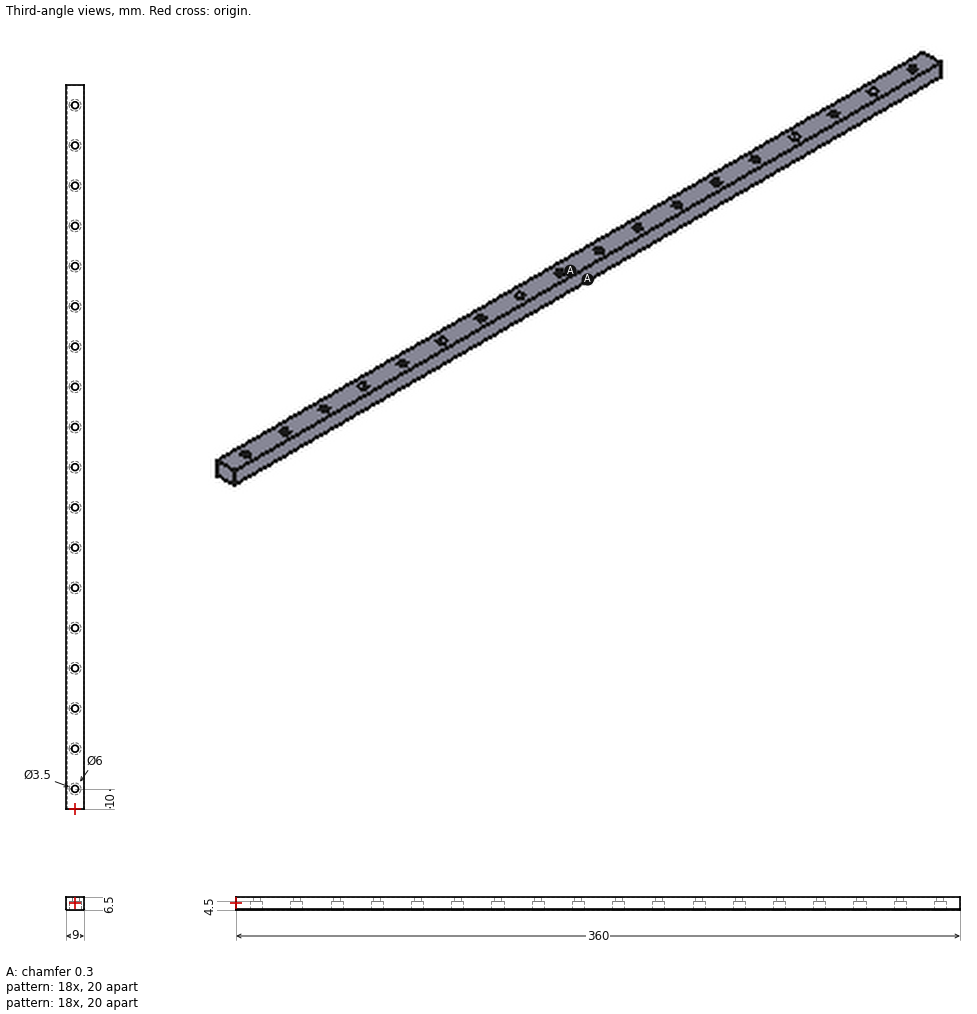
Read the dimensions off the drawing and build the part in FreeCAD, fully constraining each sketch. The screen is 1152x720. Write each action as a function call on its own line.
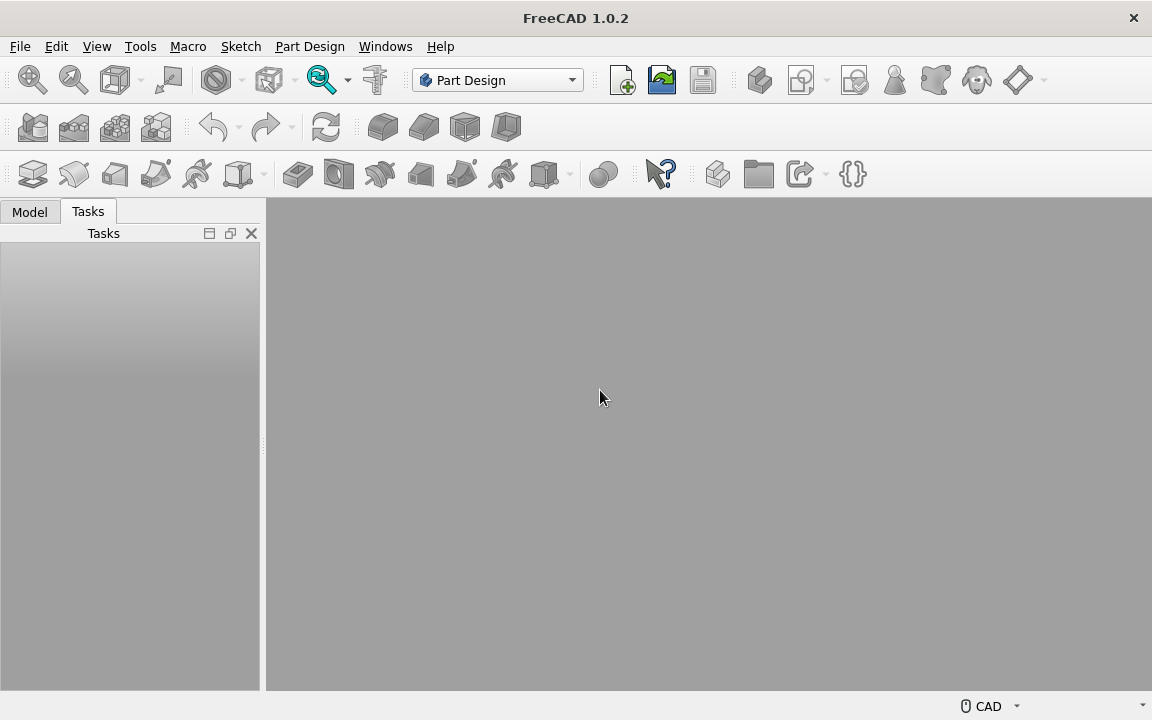
click(621, 80)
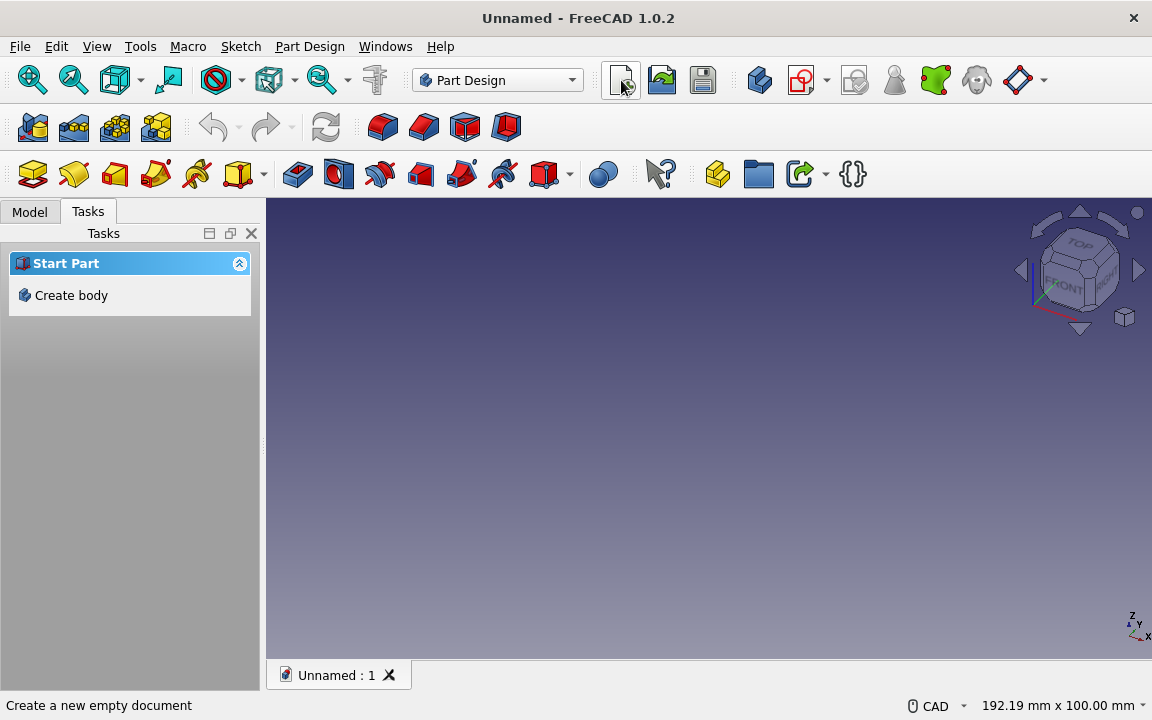
click(800, 80)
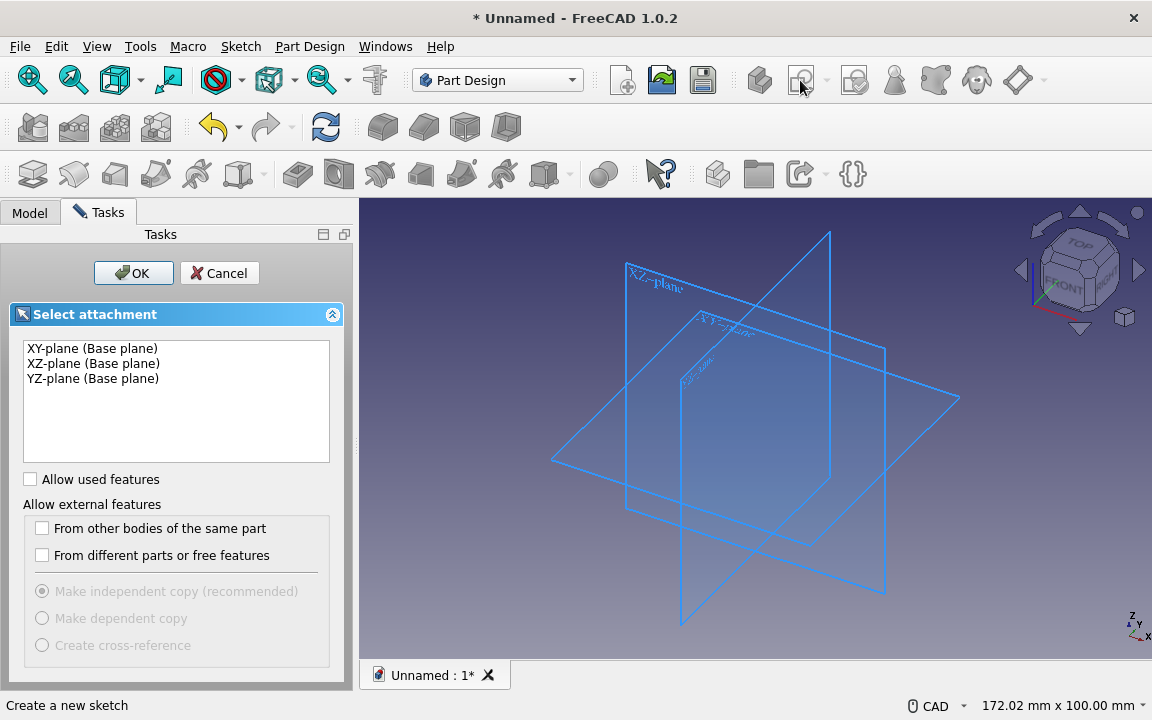
click(84, 364)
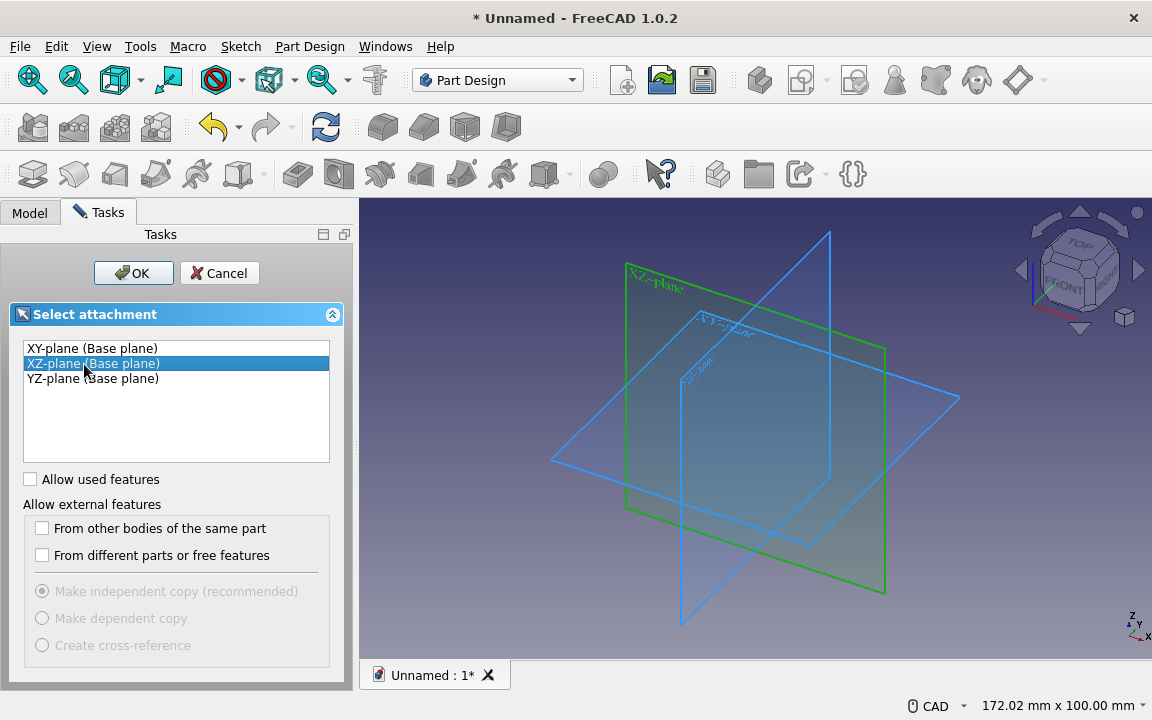
click(134, 273)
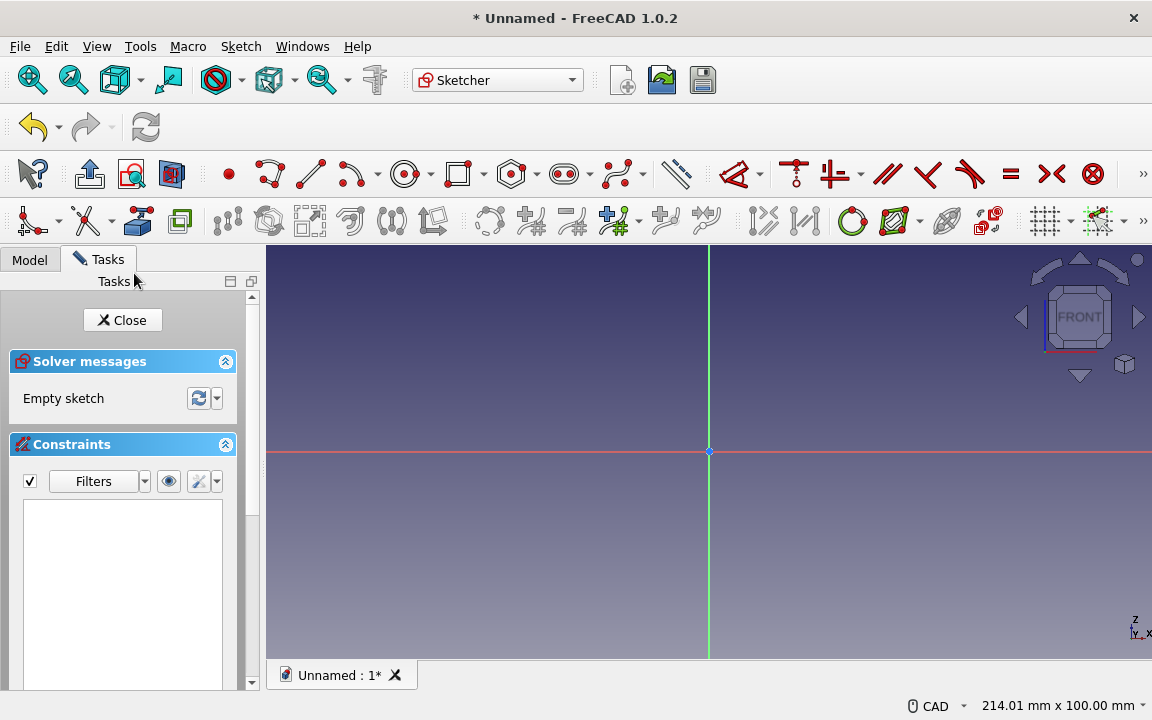
scroll(718, 452, up, 11)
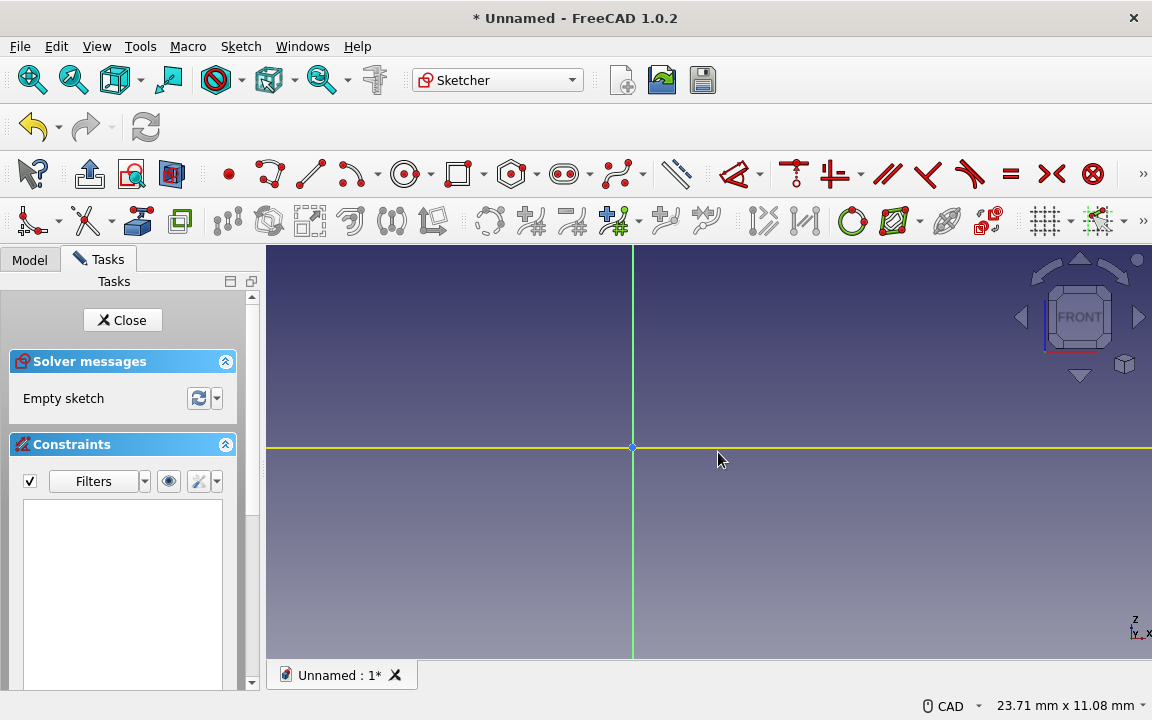
key(g)
key(v)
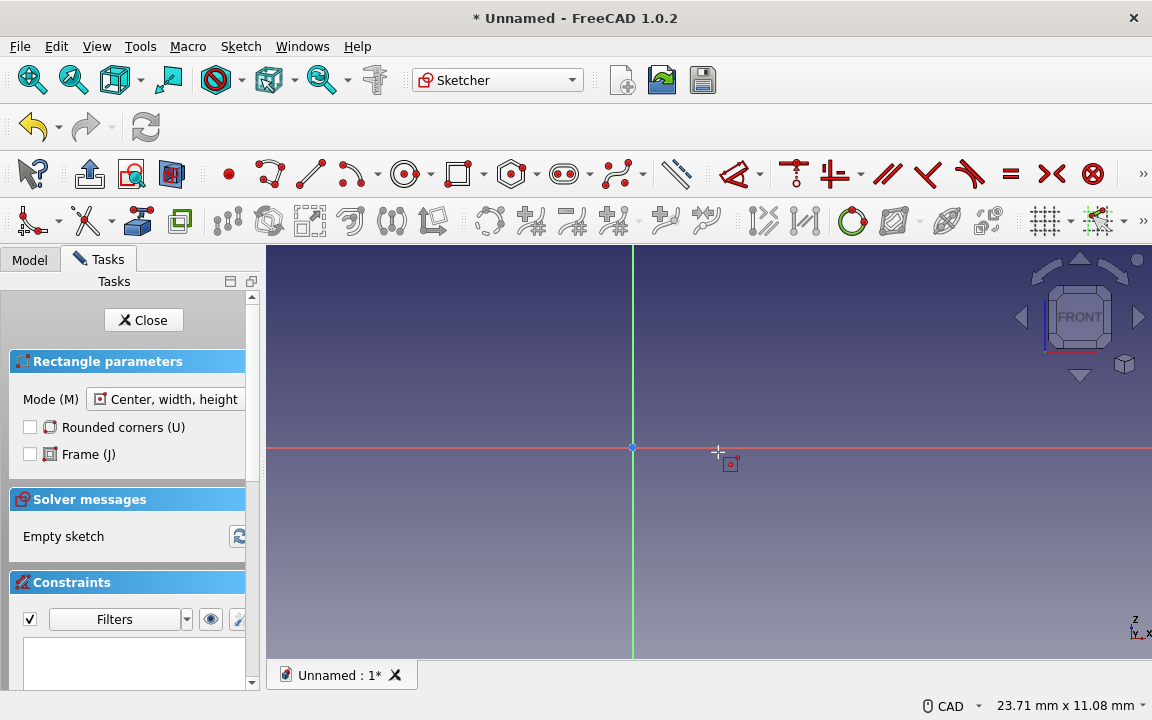
click(633, 448)
move(801, 327)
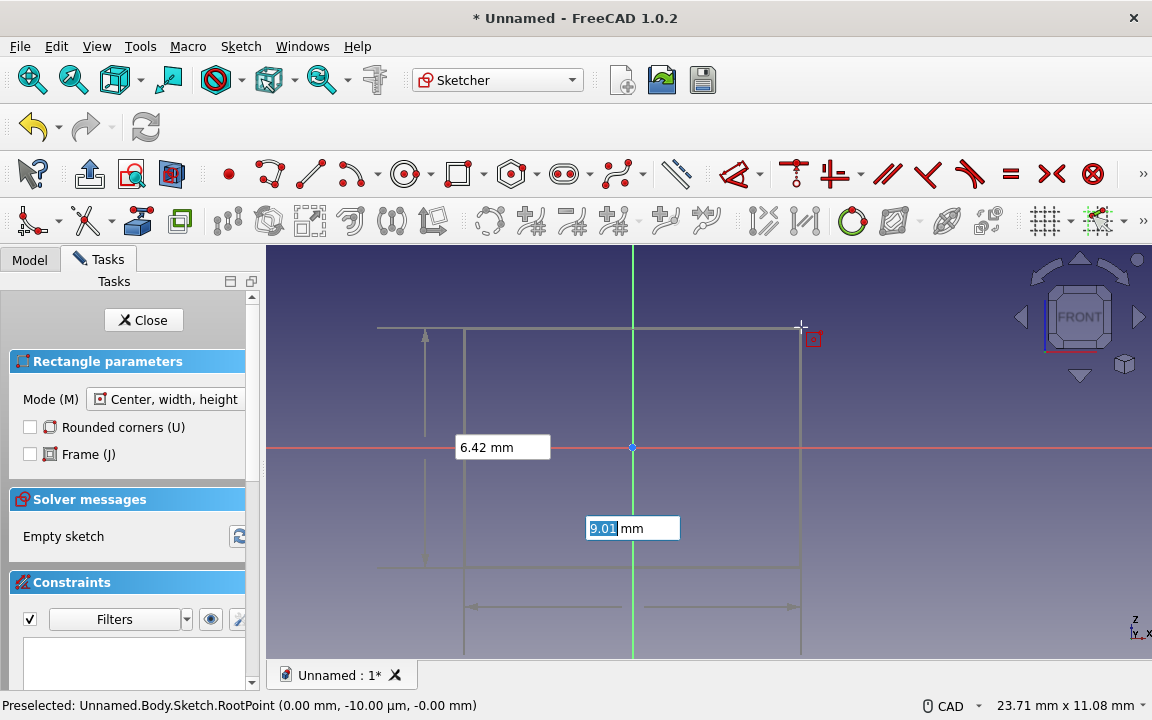
text(9)
key(Tab)
text(6.5)
key(Return)
key(Escape)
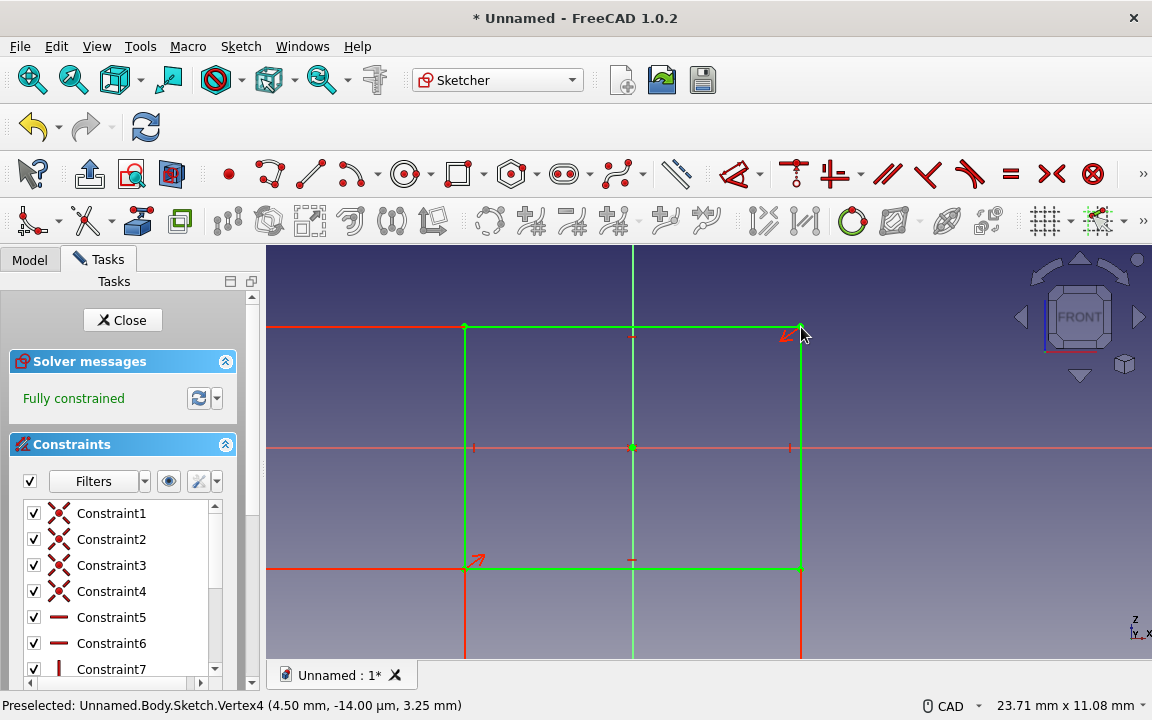
click(123, 320)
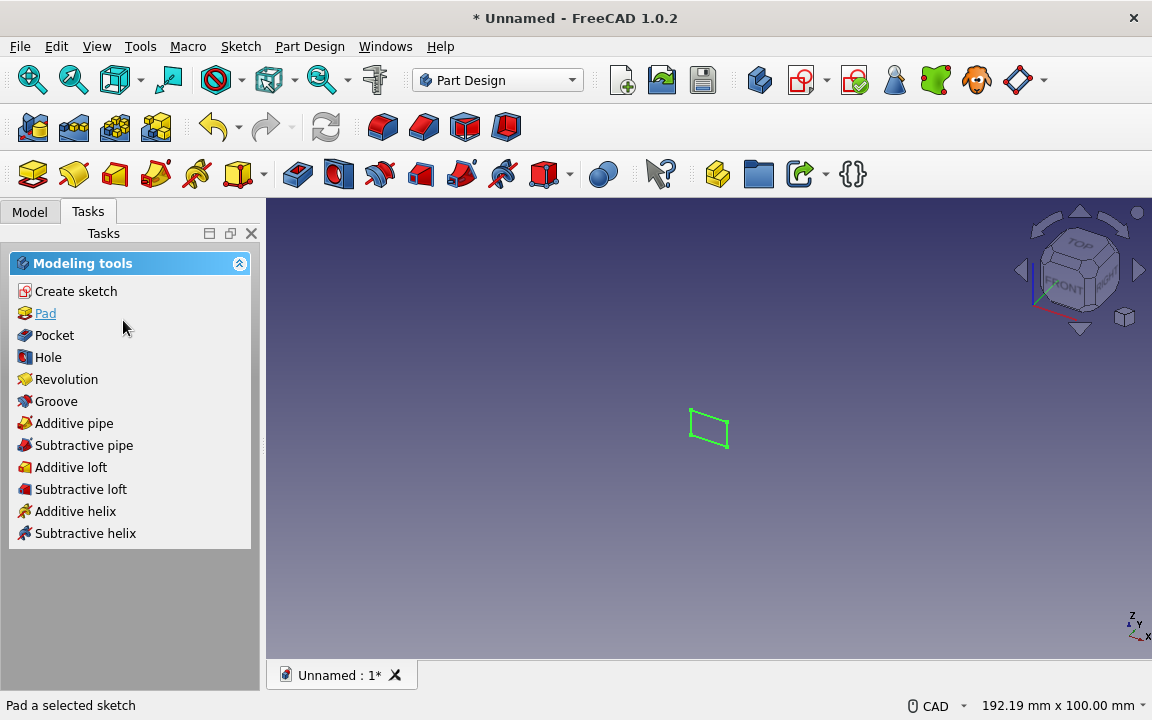
click(33, 174)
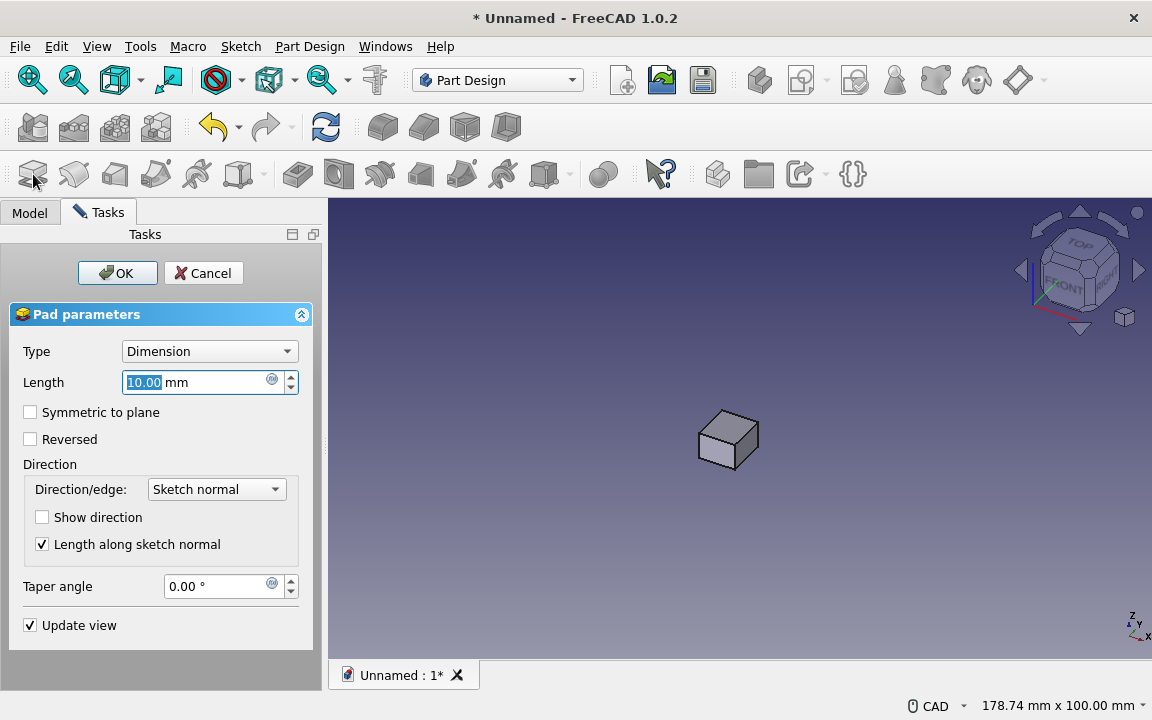
text(360)
key(Tab)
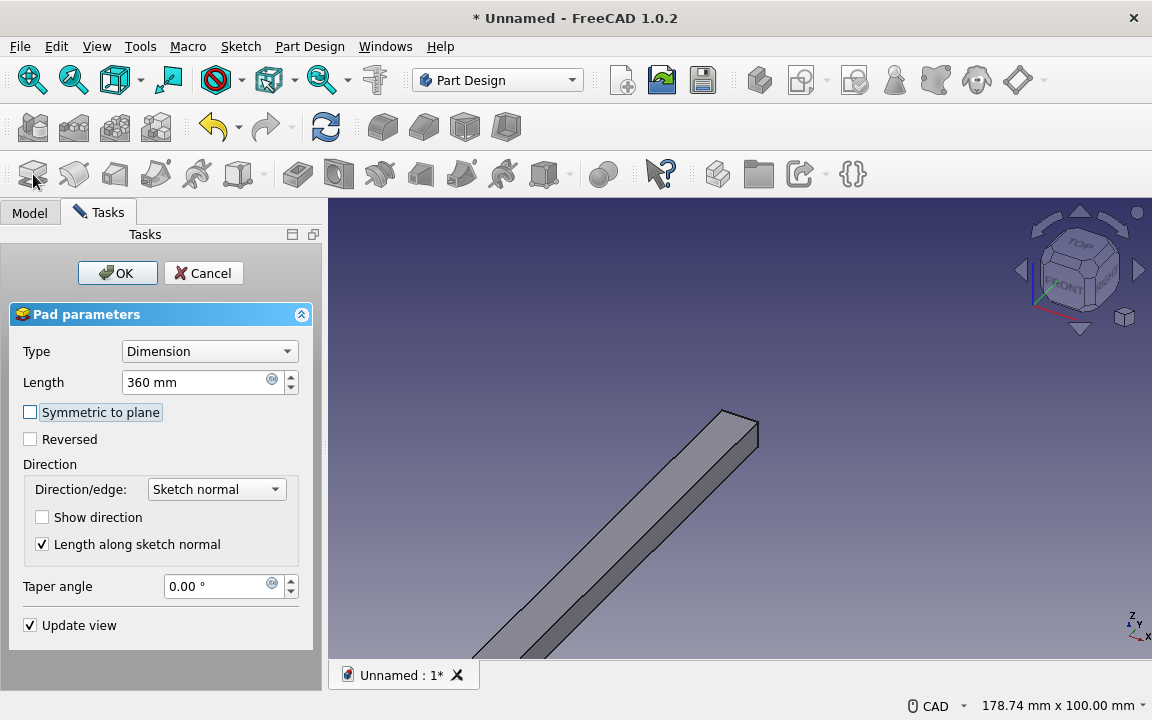
click(31, 439)